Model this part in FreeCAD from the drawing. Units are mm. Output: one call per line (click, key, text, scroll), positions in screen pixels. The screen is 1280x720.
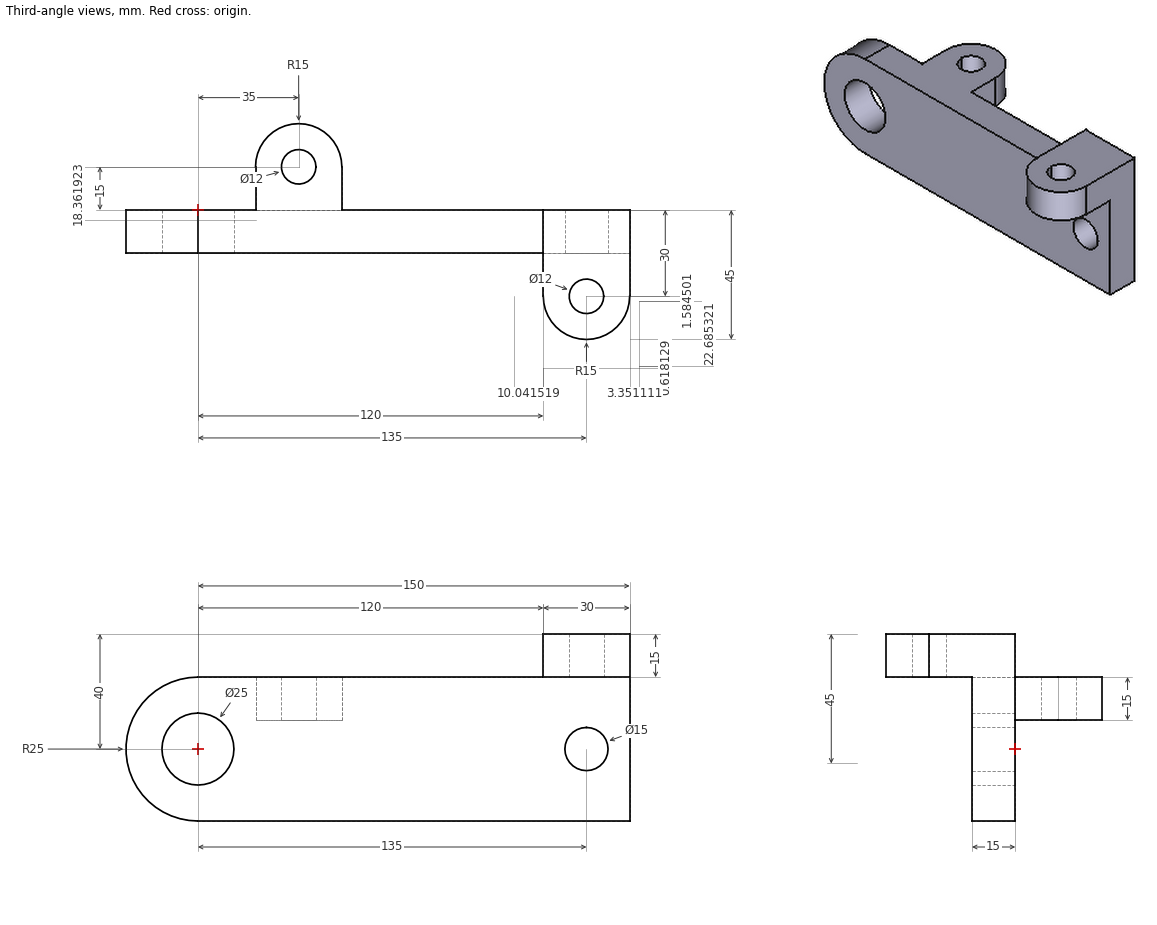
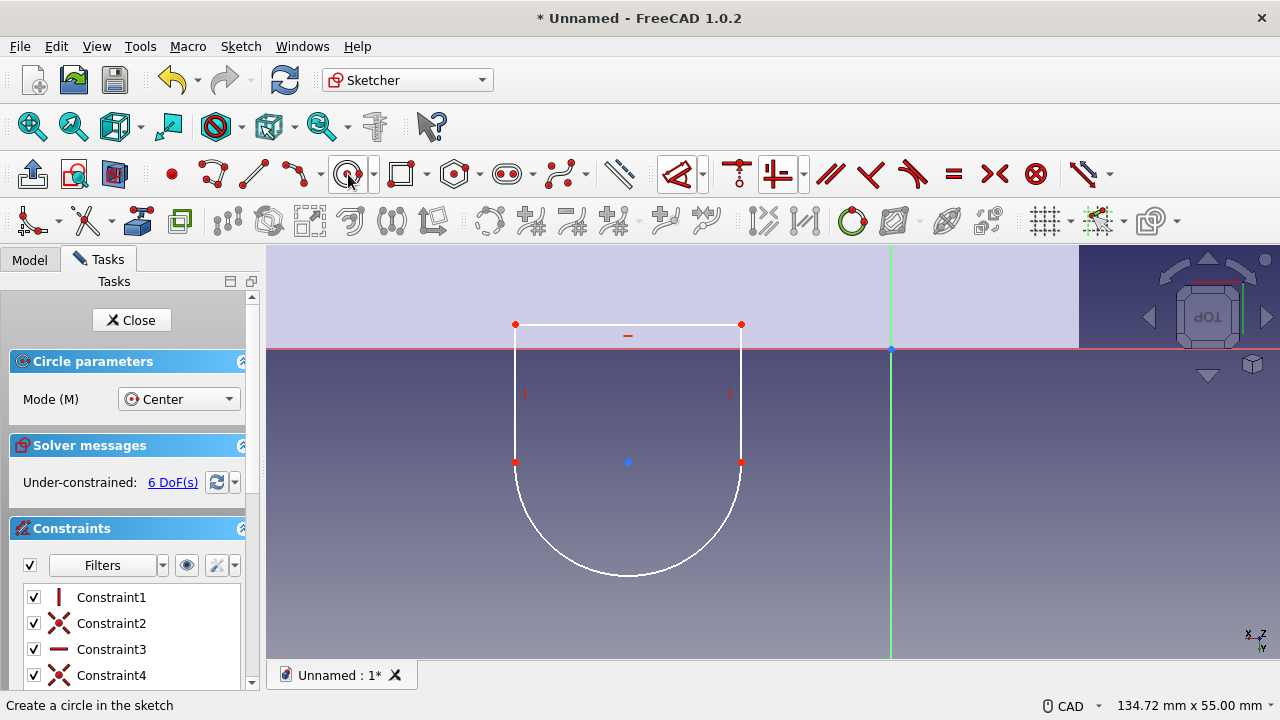
click(628, 462)
click(660, 430)
key(Escape)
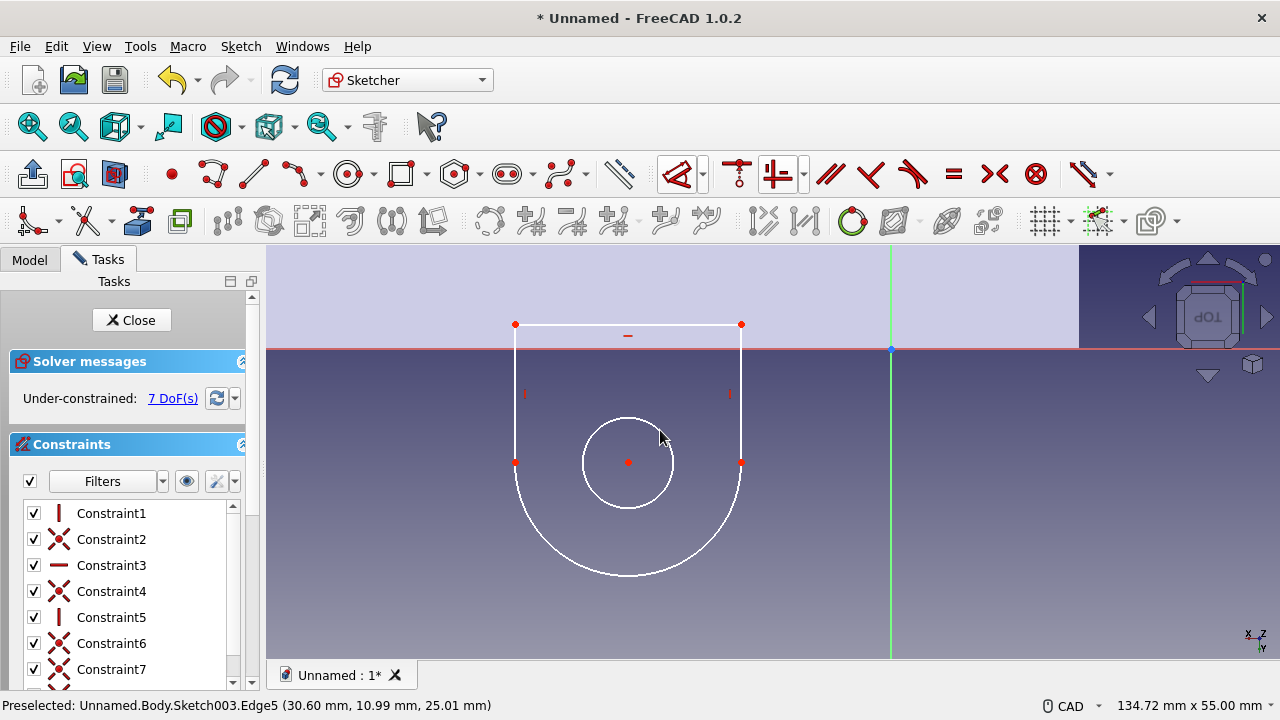
click(741, 422)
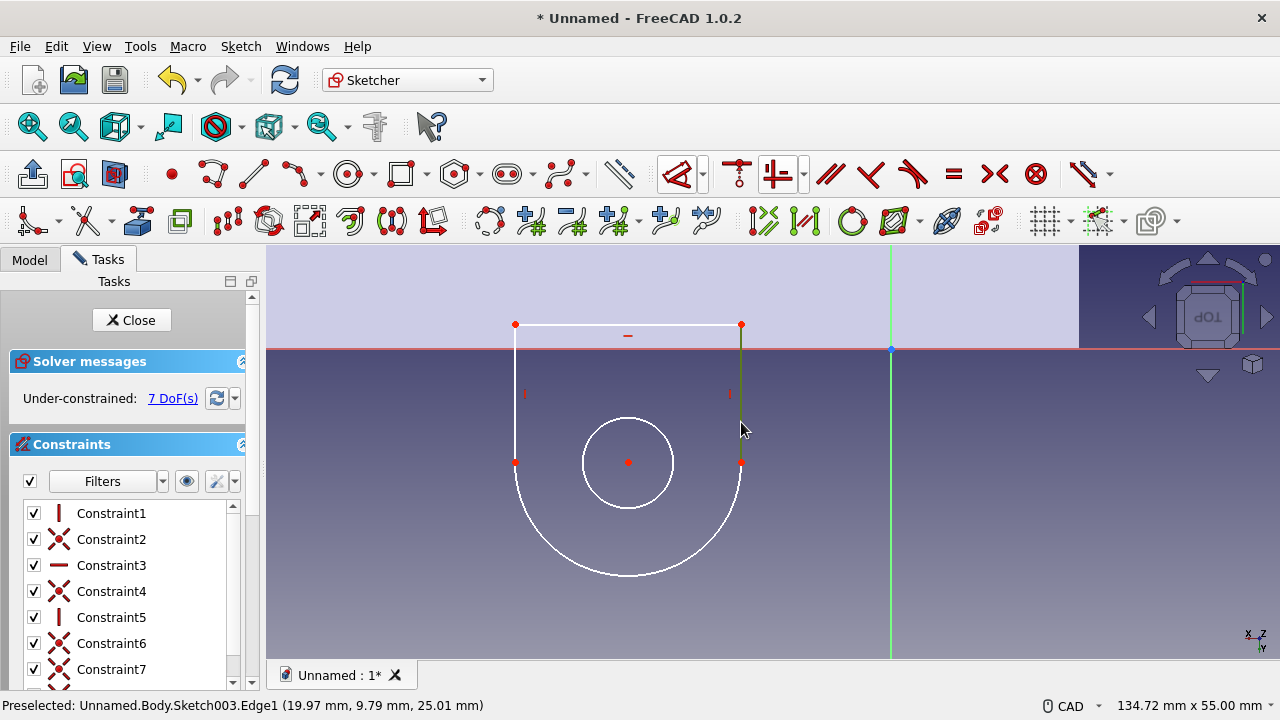
click(562, 554)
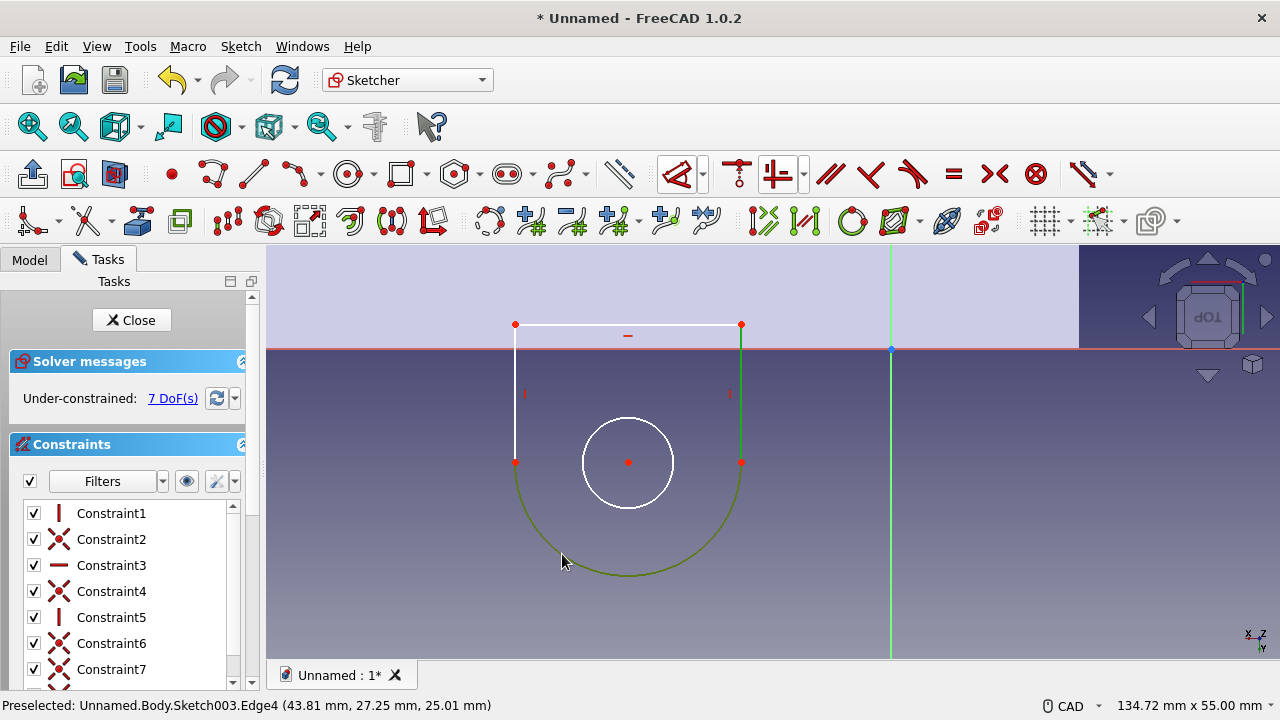
click(913, 174)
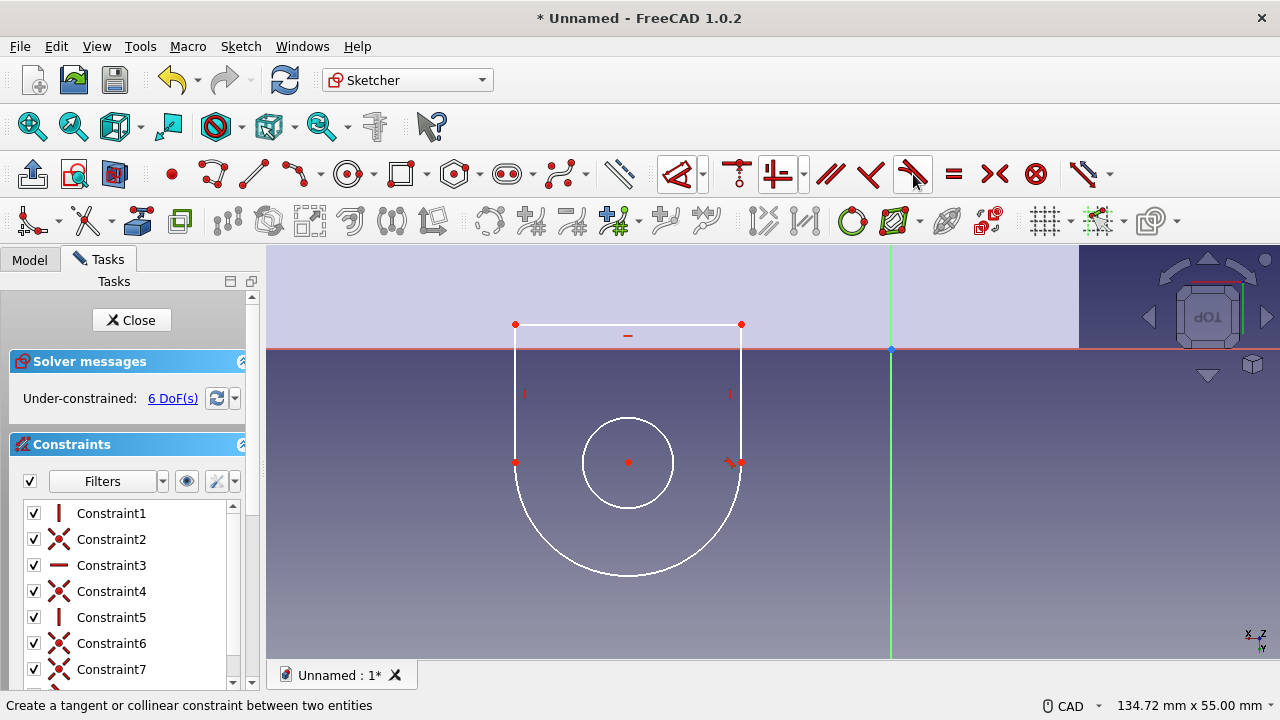
click(515, 366)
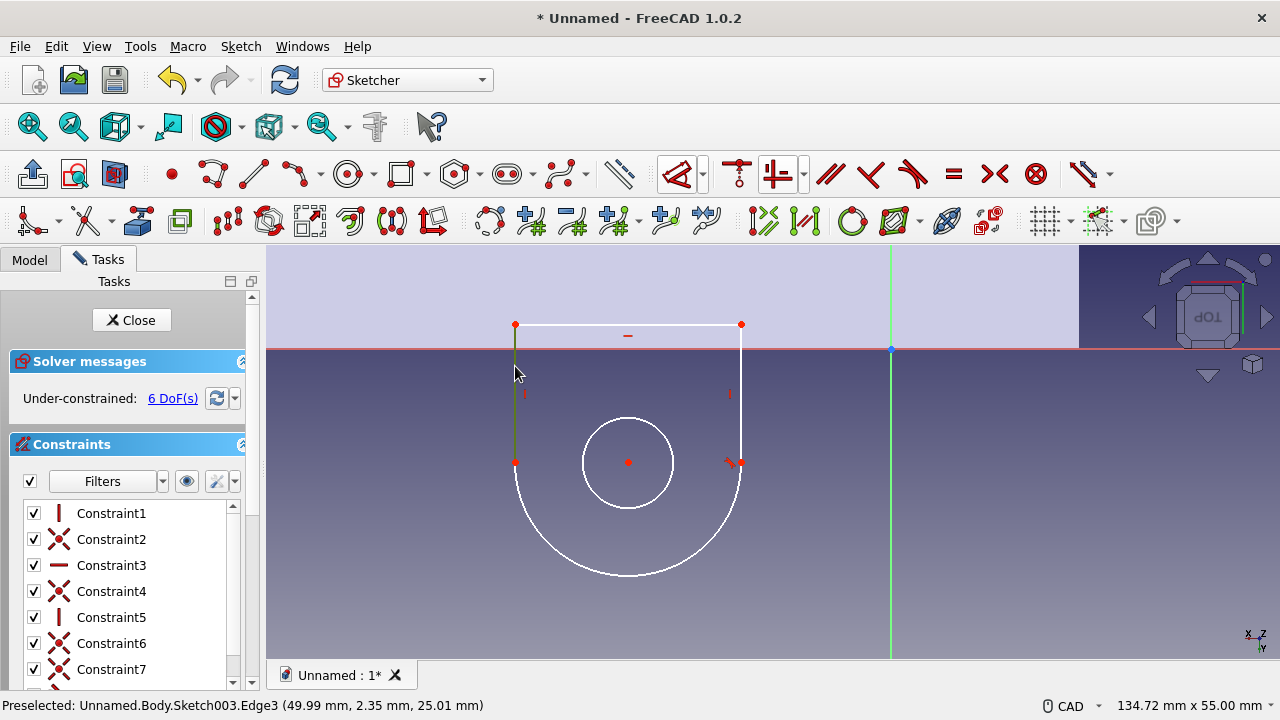
click(562, 554)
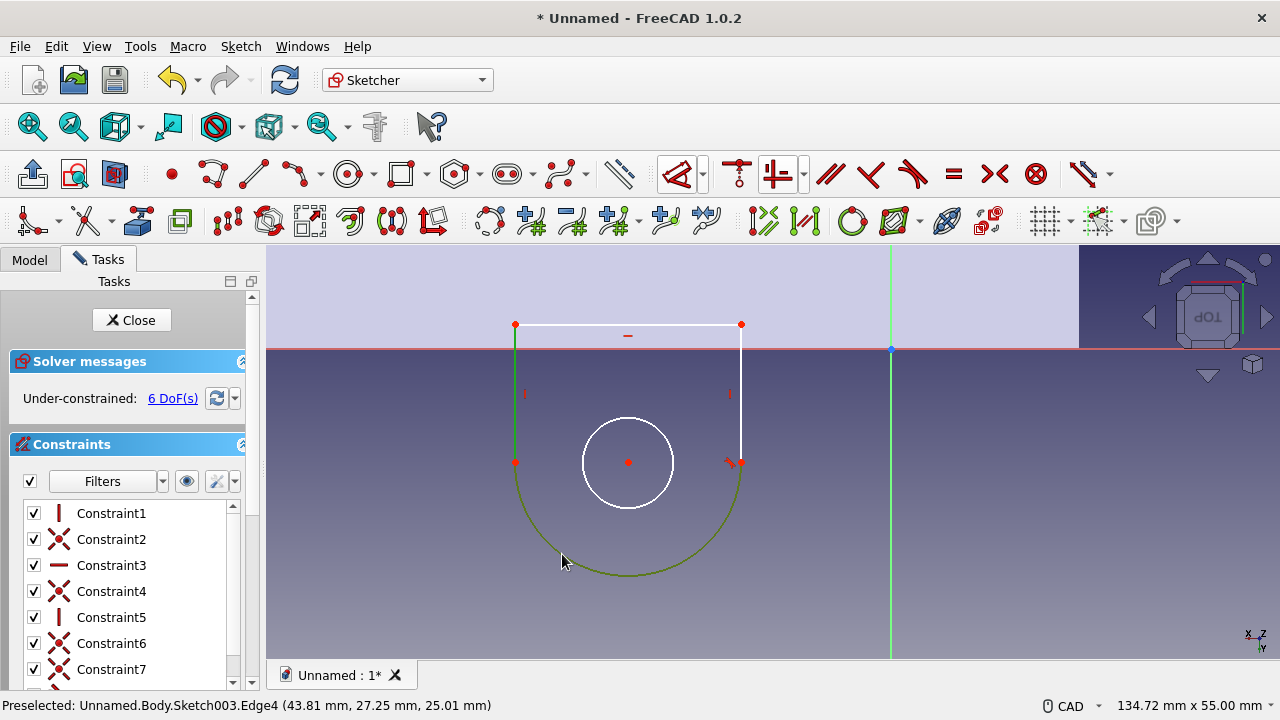
click(913, 174)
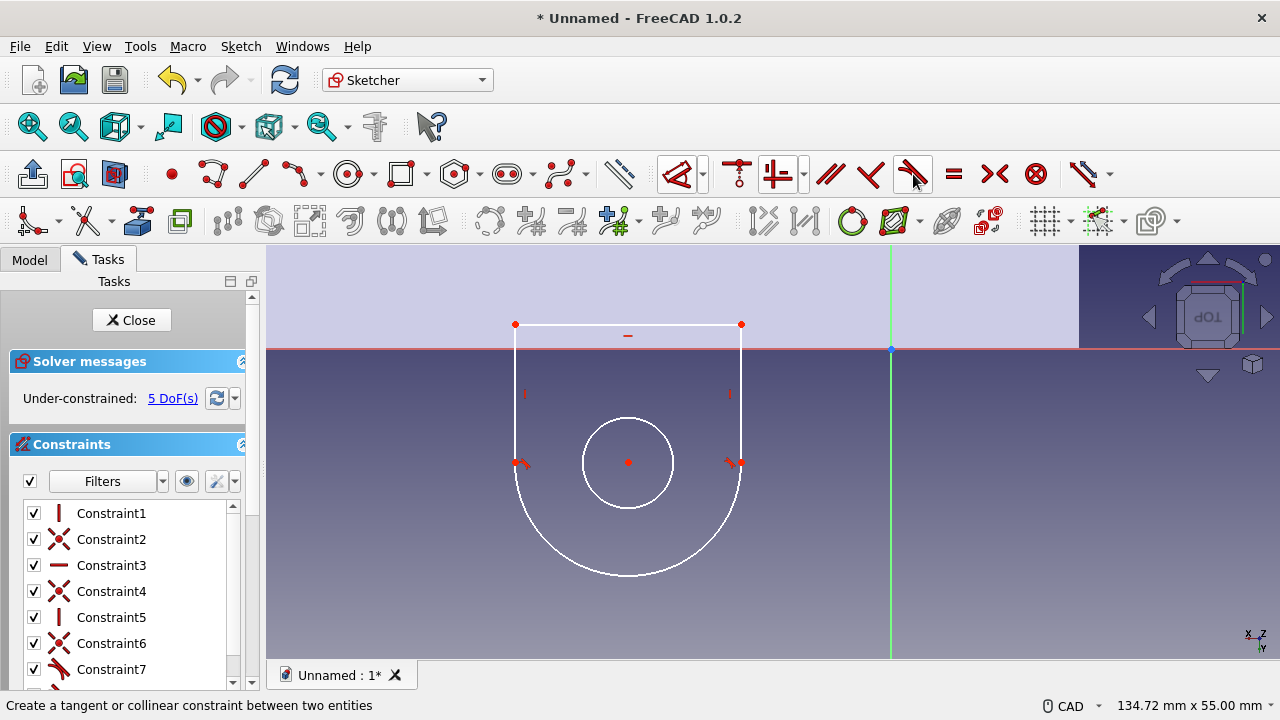
click(562, 554)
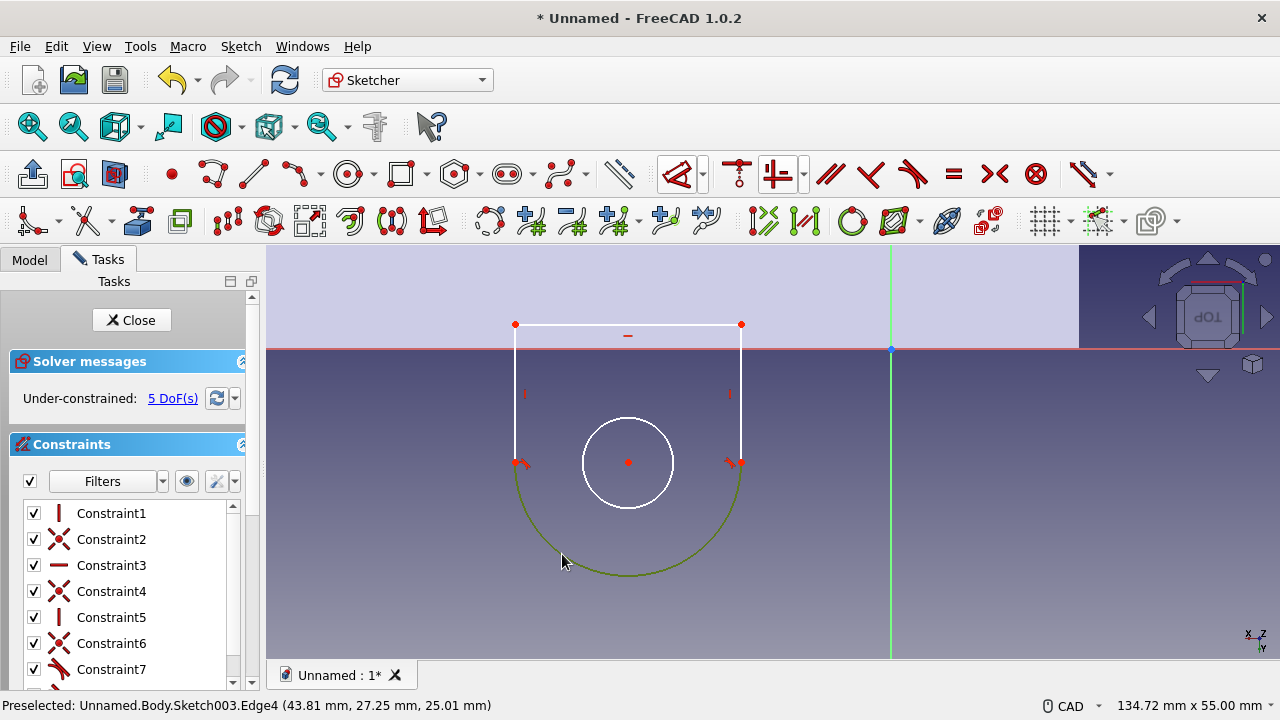
click(702, 174)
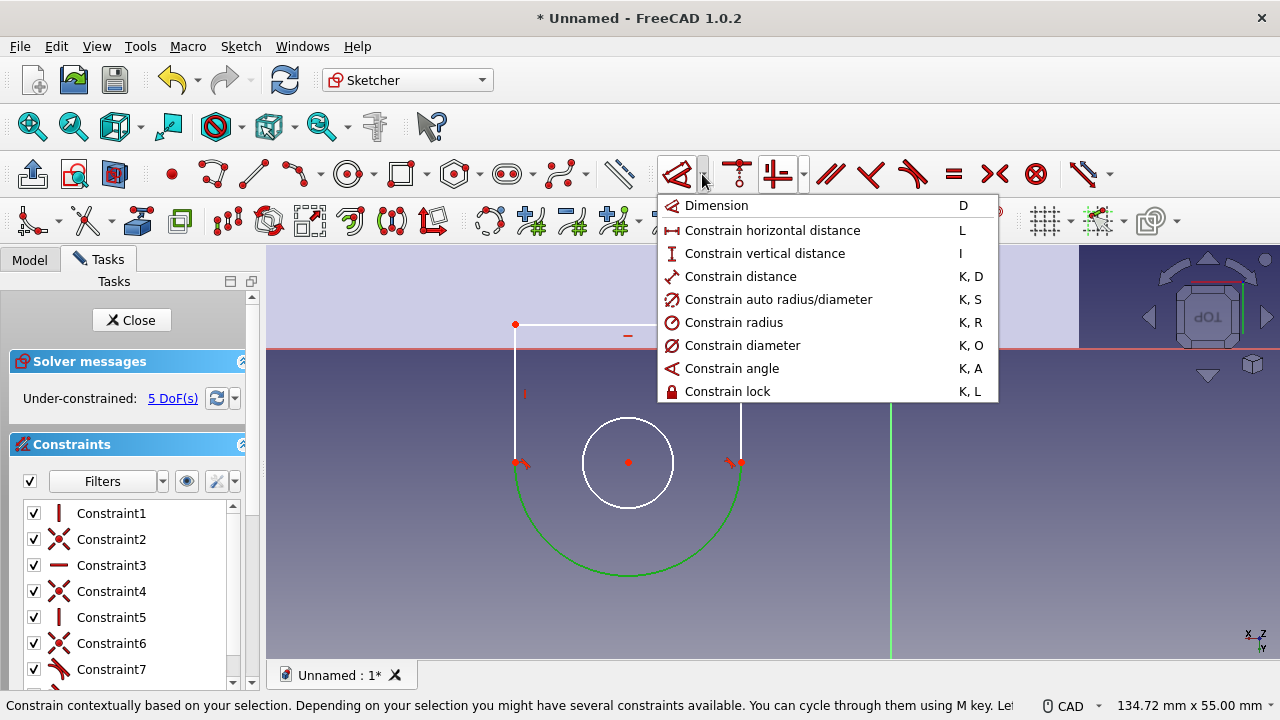
click(828, 322)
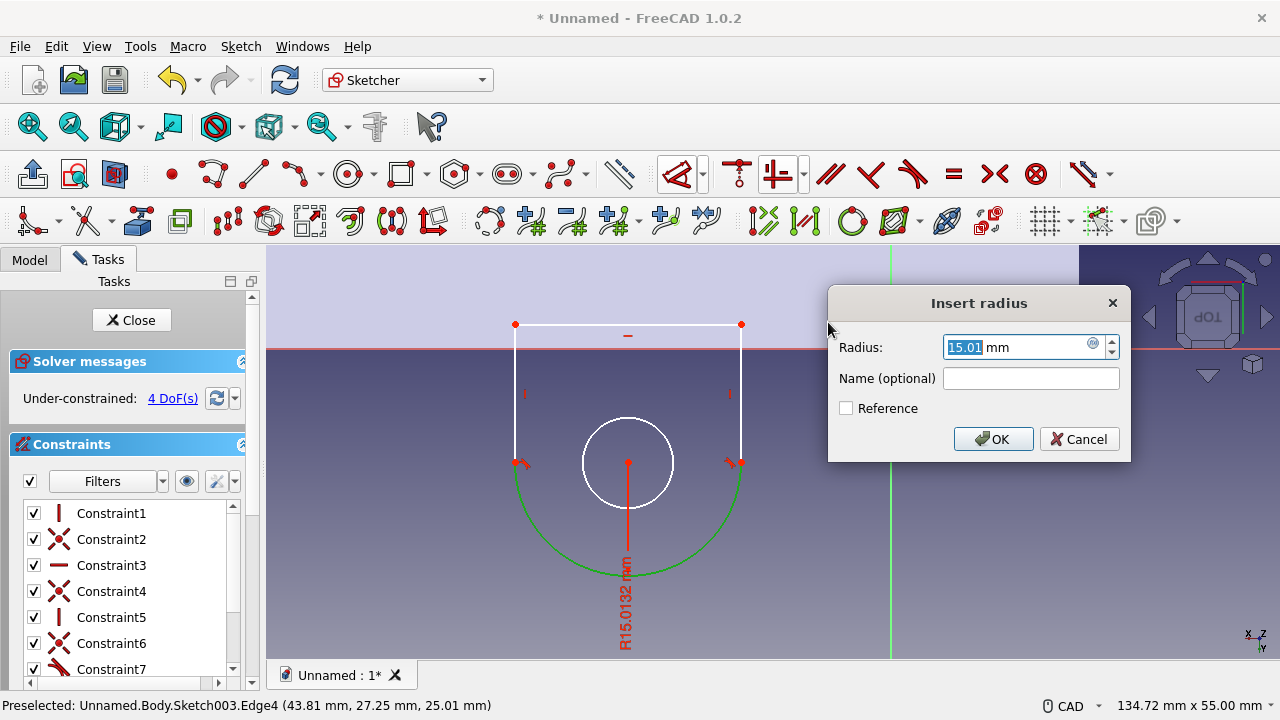
text(15)
key(Return)